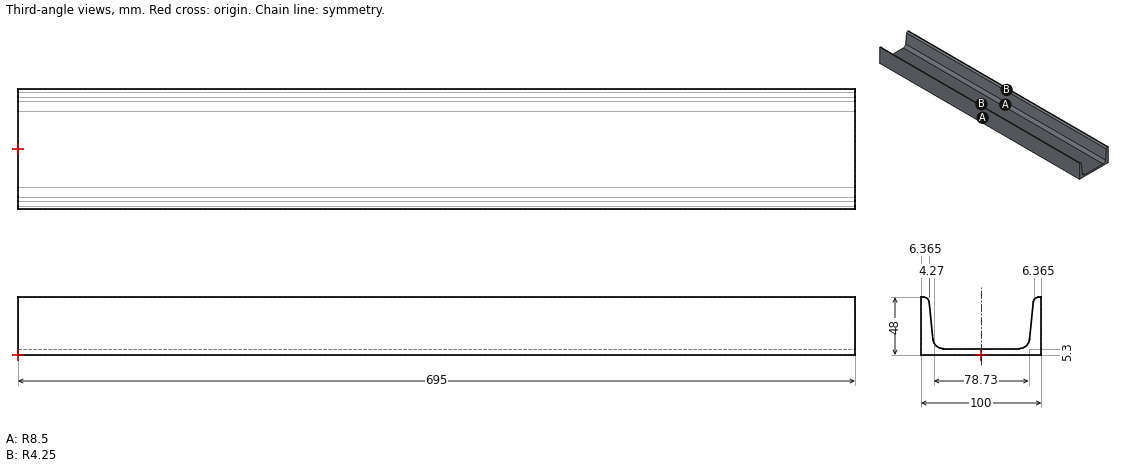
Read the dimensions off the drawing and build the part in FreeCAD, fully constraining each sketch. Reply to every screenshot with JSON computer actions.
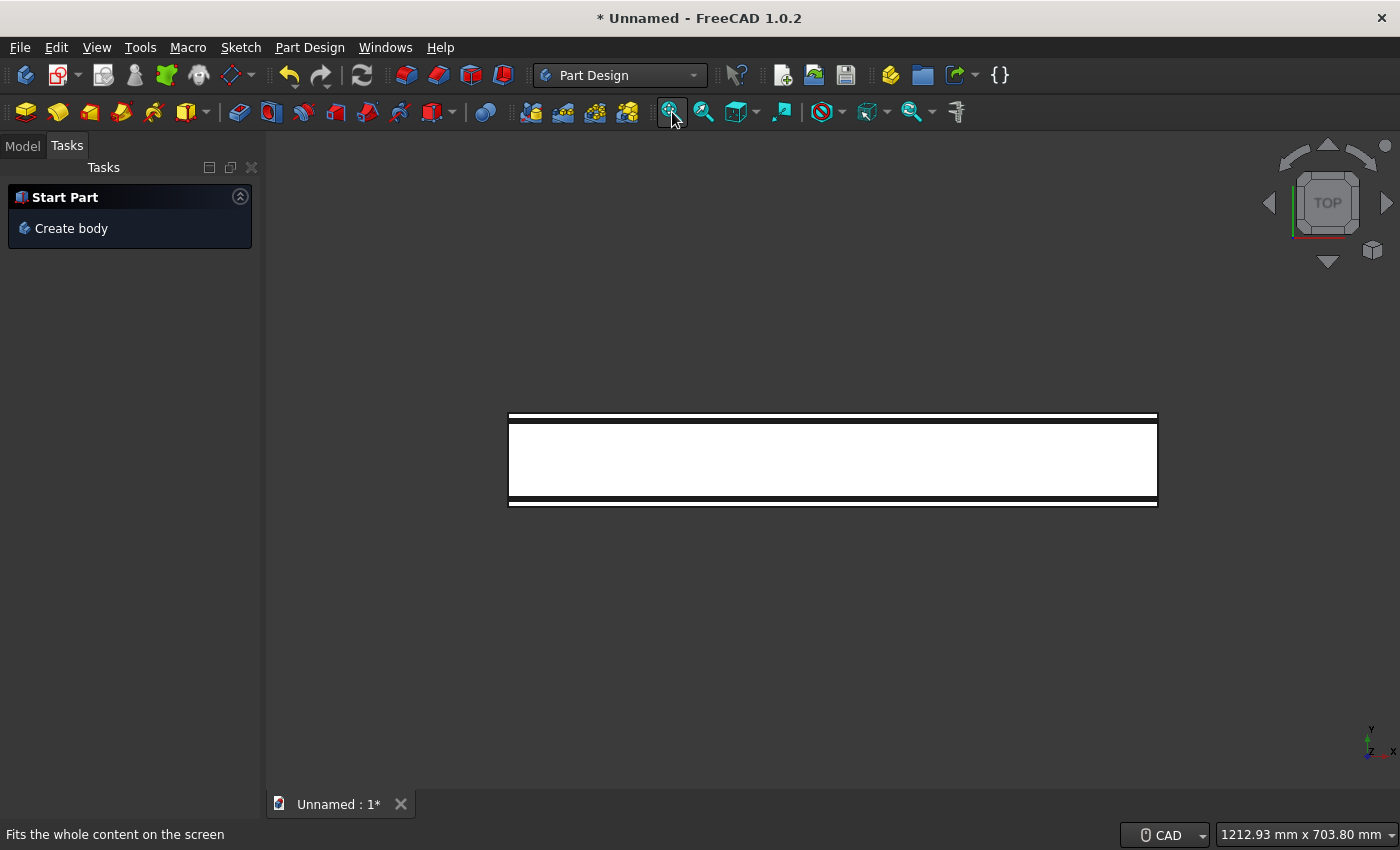
{"action": "key", "text": "1"}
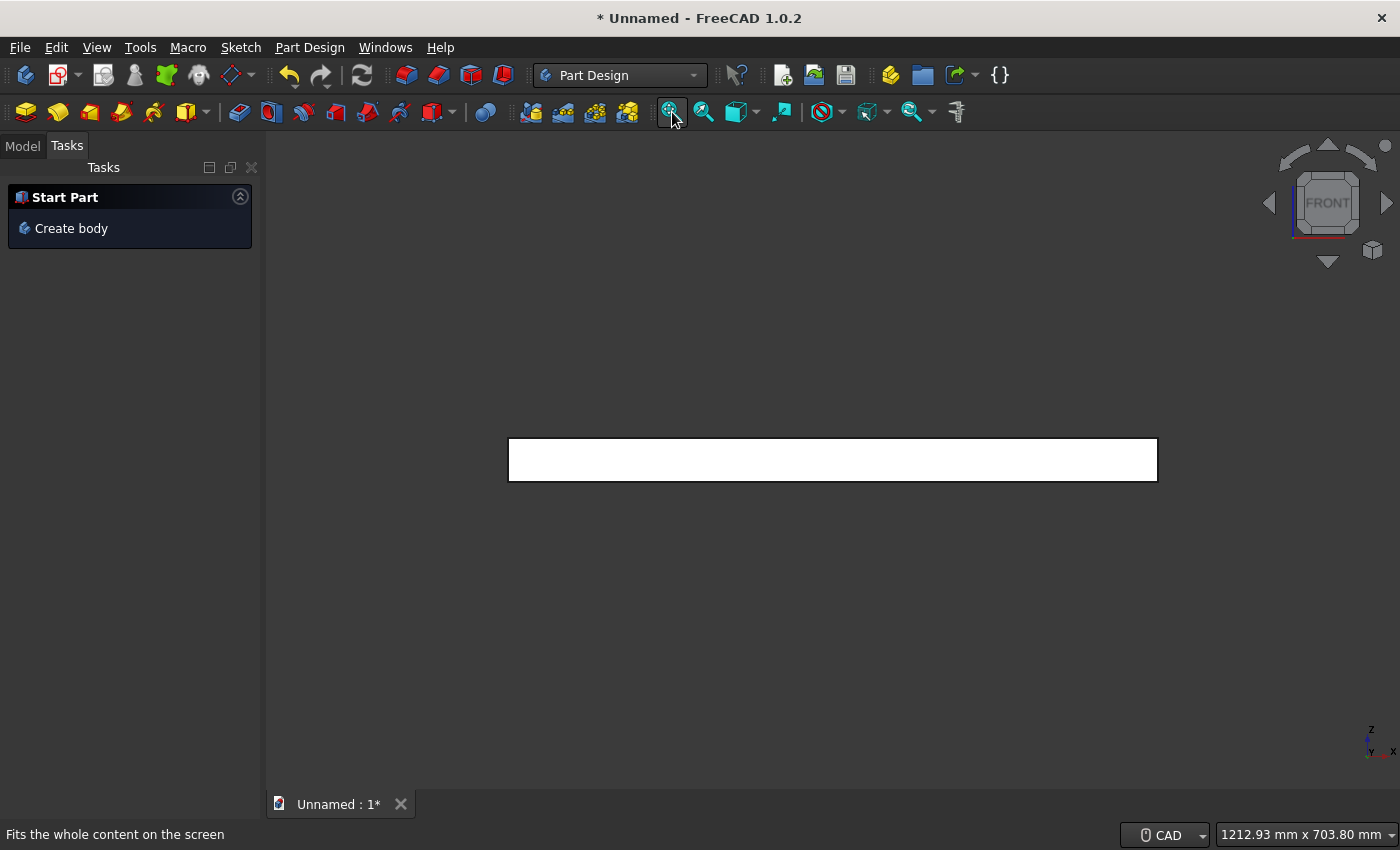
{"action": "key", "text": "3"}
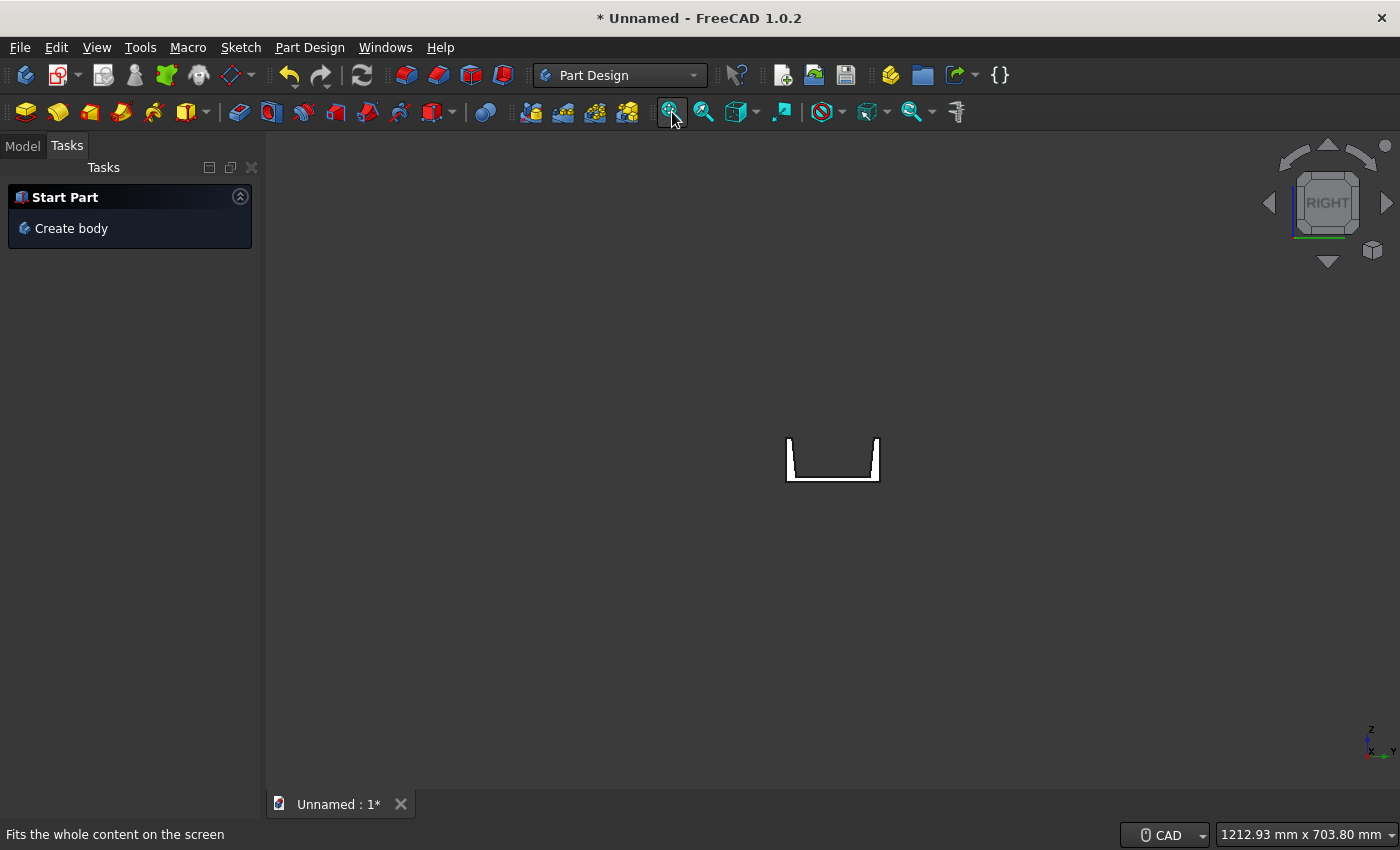
{"action": "left_click", "coordinate": [672, 112]}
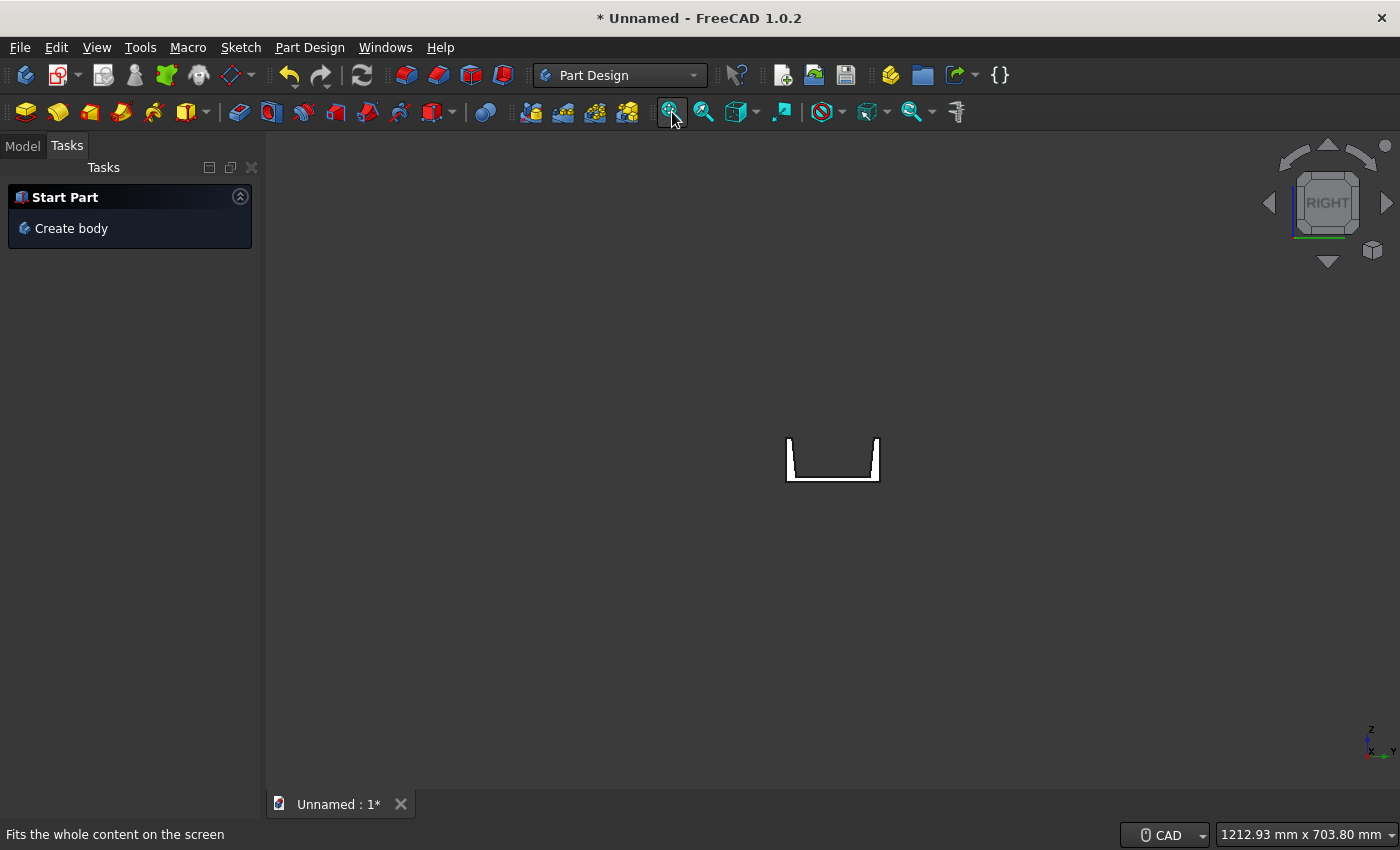
{"action": "key", "text": "5"}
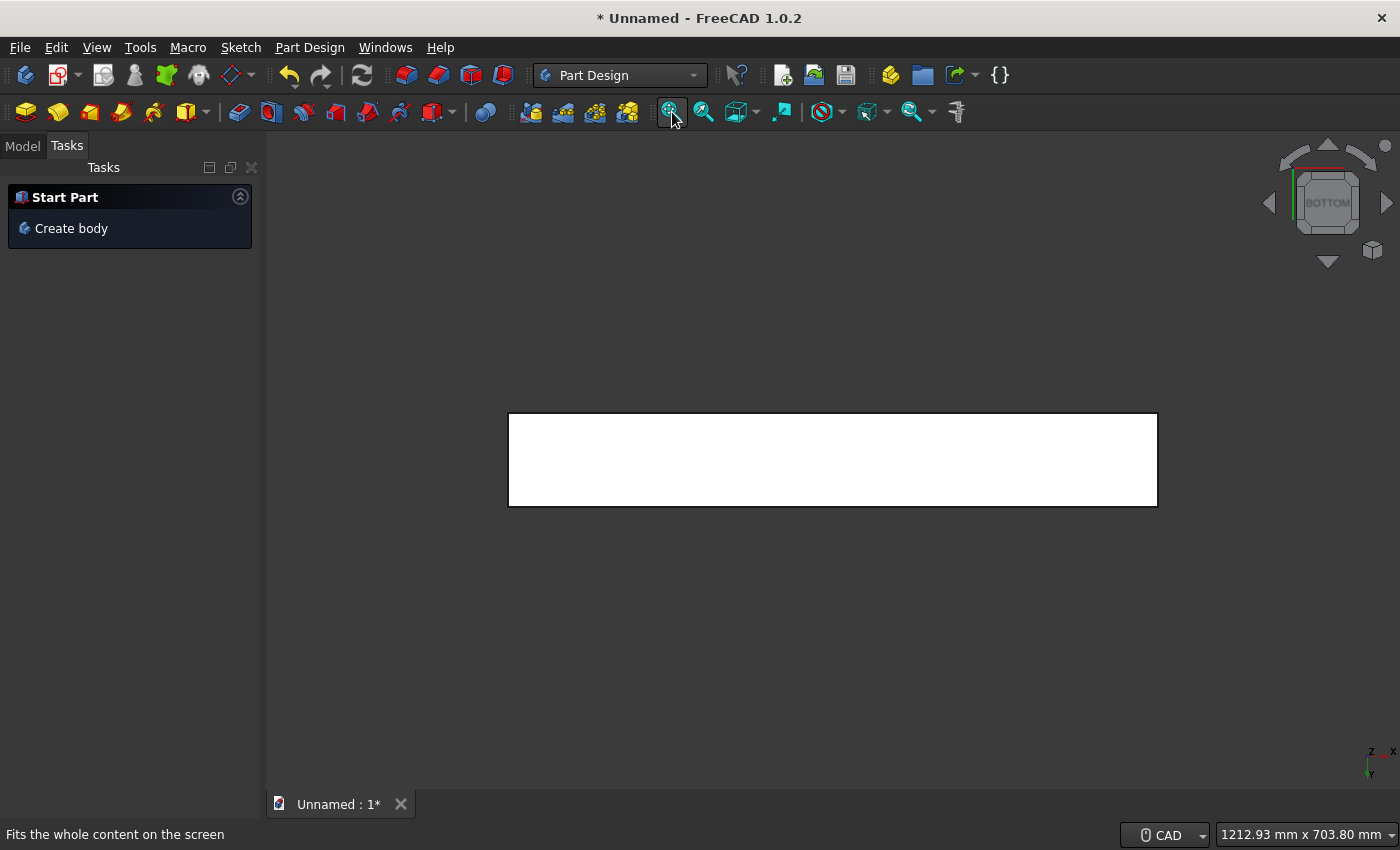
{"action": "key", "text": "4"}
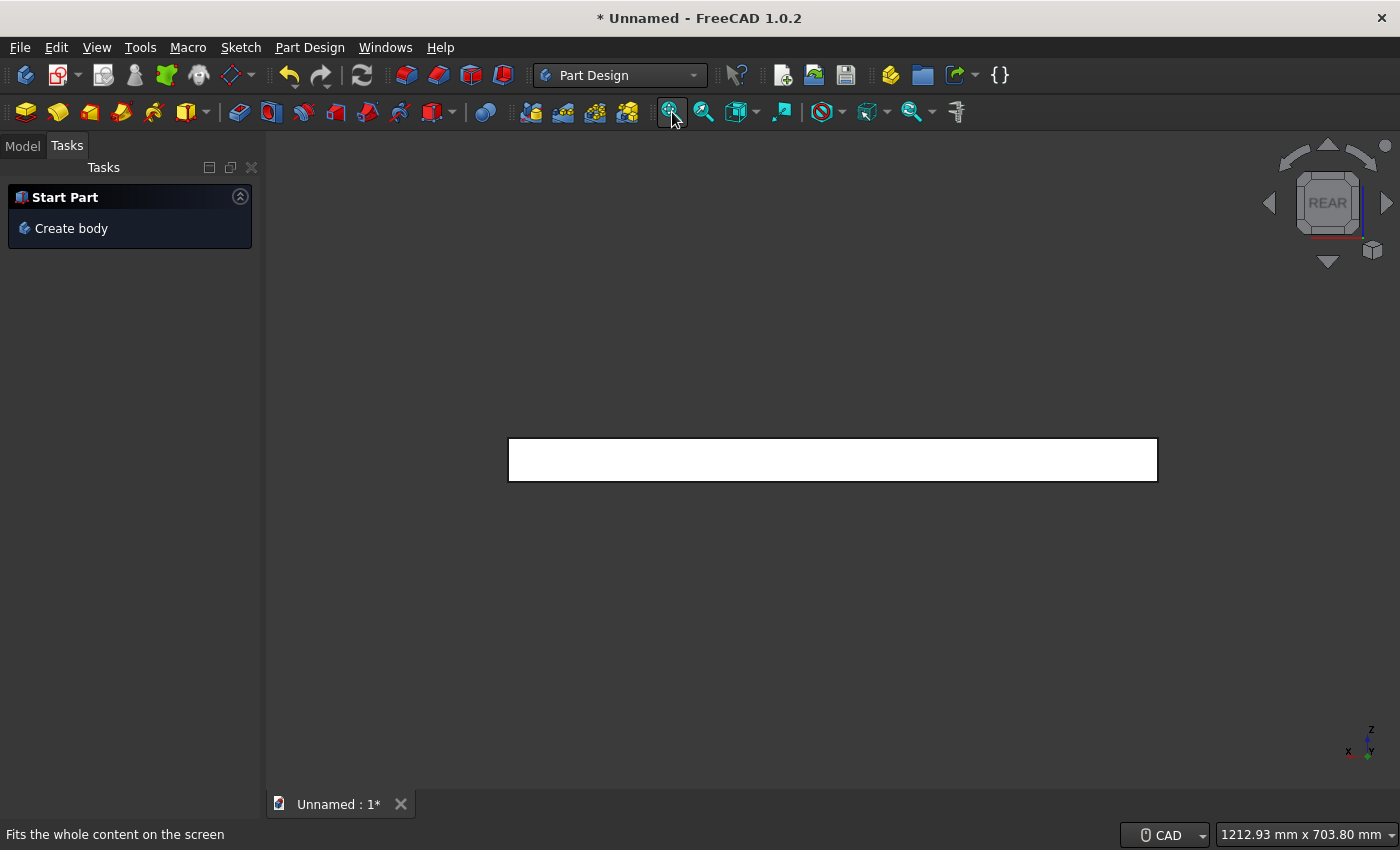
{"action": "key", "text": "6"}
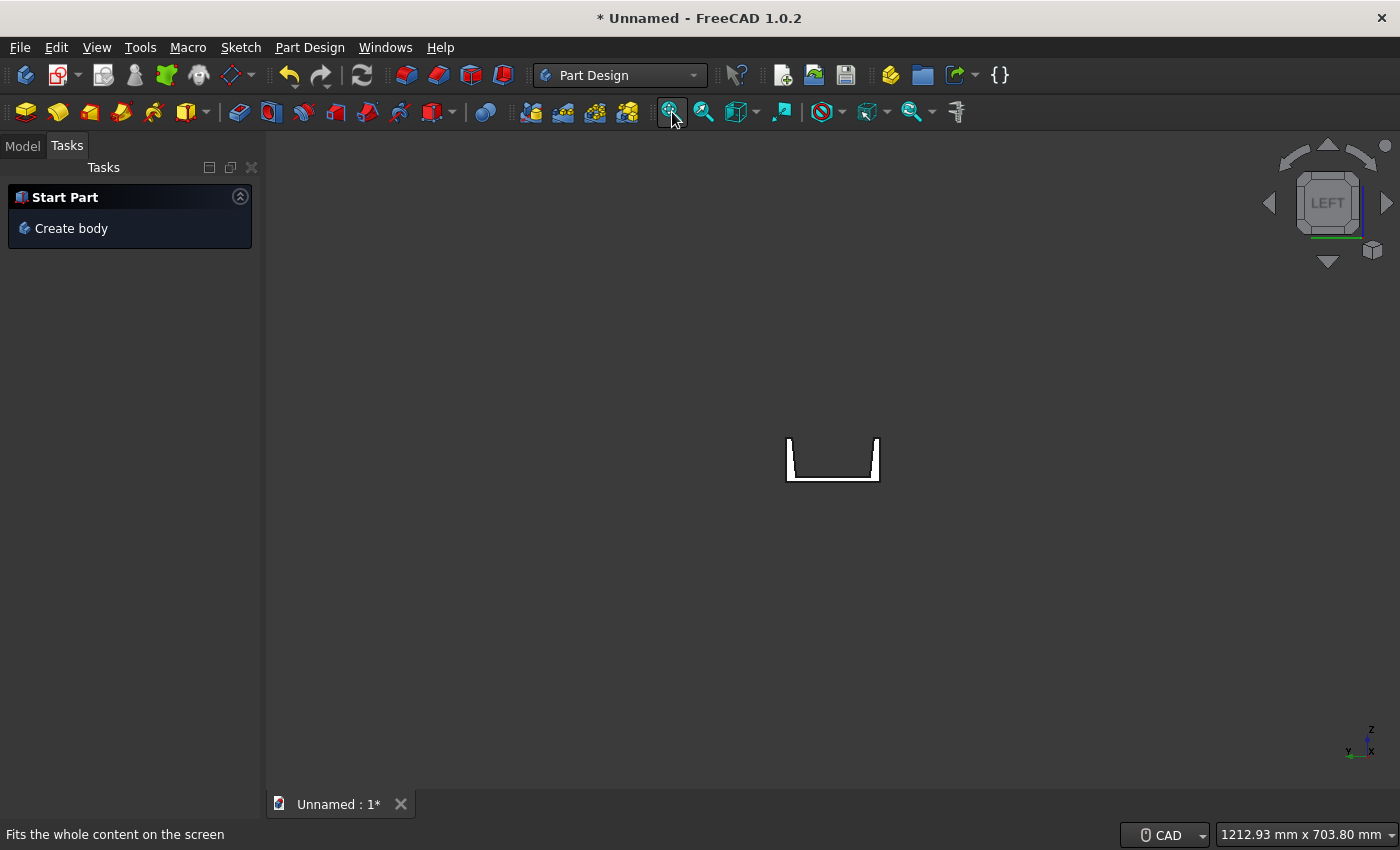
{"action": "left_click", "coordinate": [672, 112]}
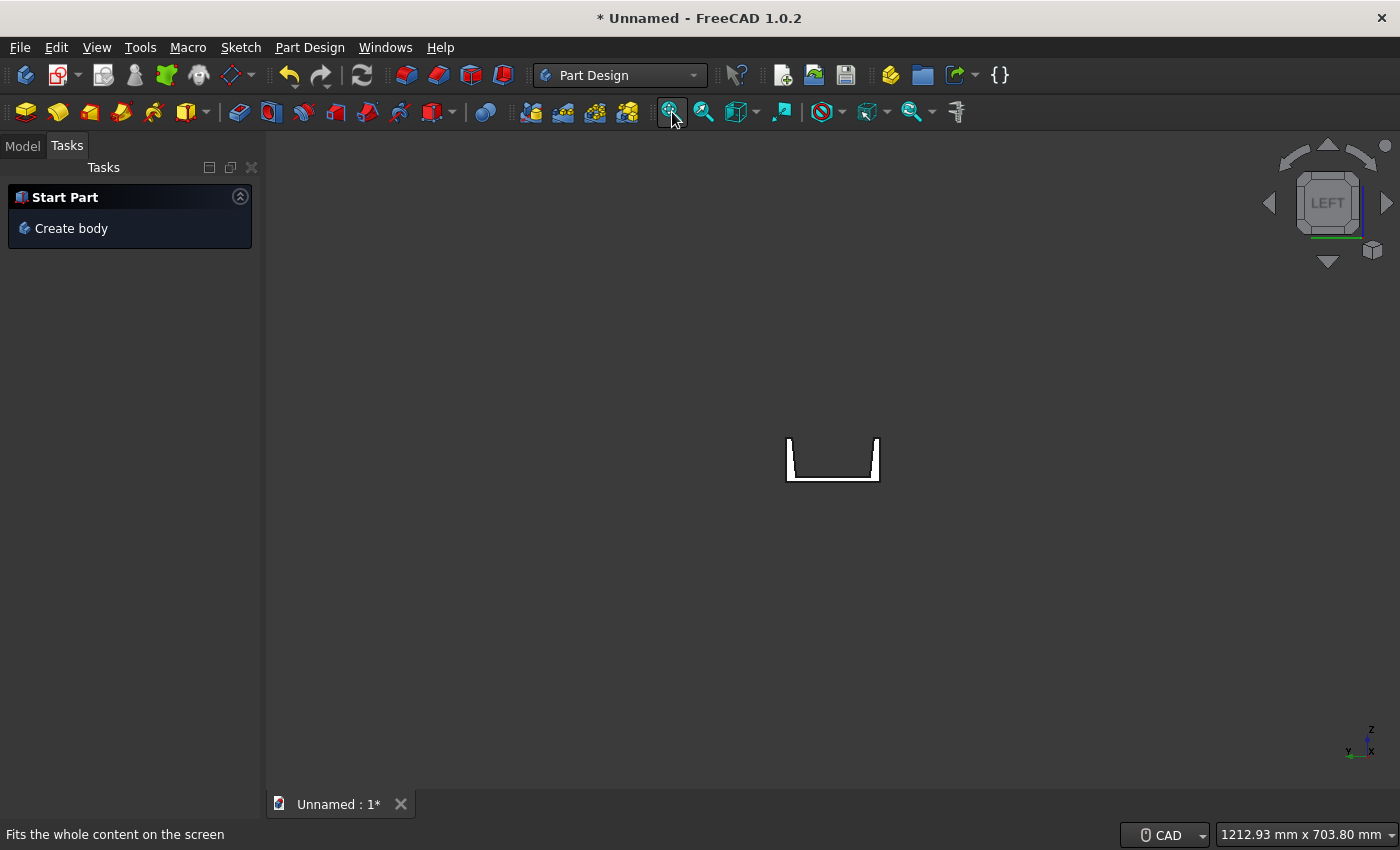
{"action": "key", "text": "v 3"}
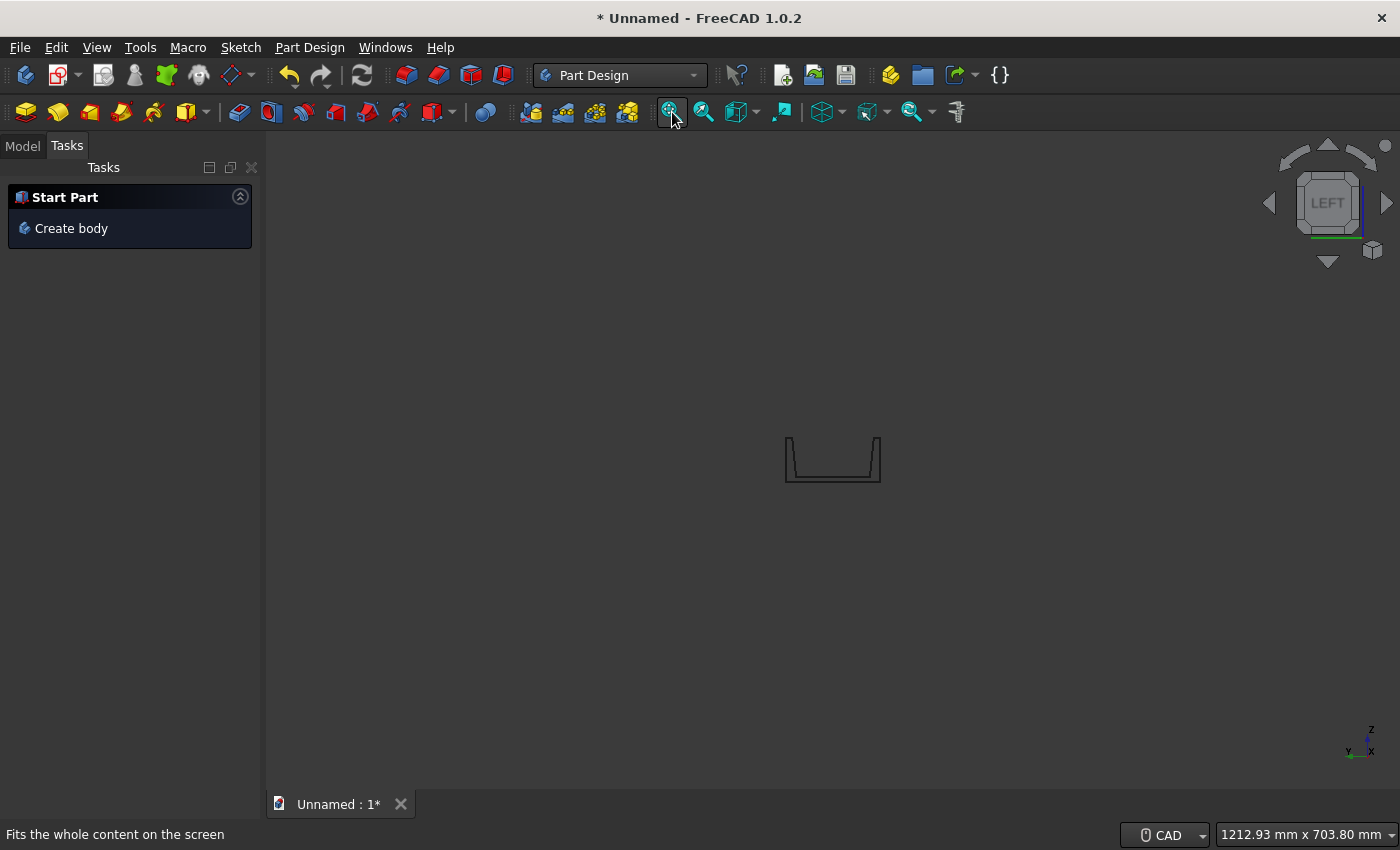
{"action": "key", "text": "0"}